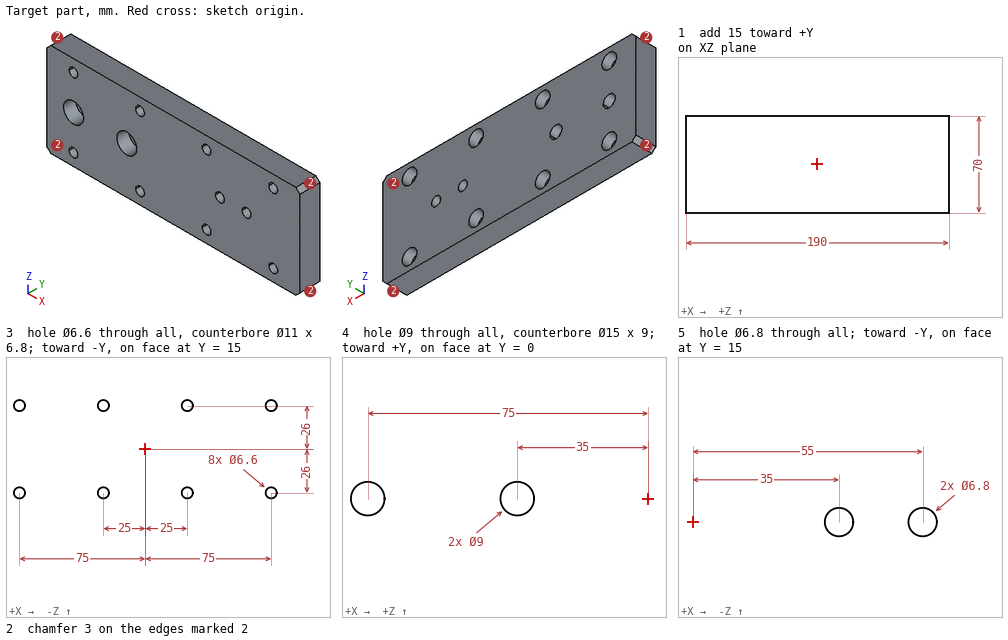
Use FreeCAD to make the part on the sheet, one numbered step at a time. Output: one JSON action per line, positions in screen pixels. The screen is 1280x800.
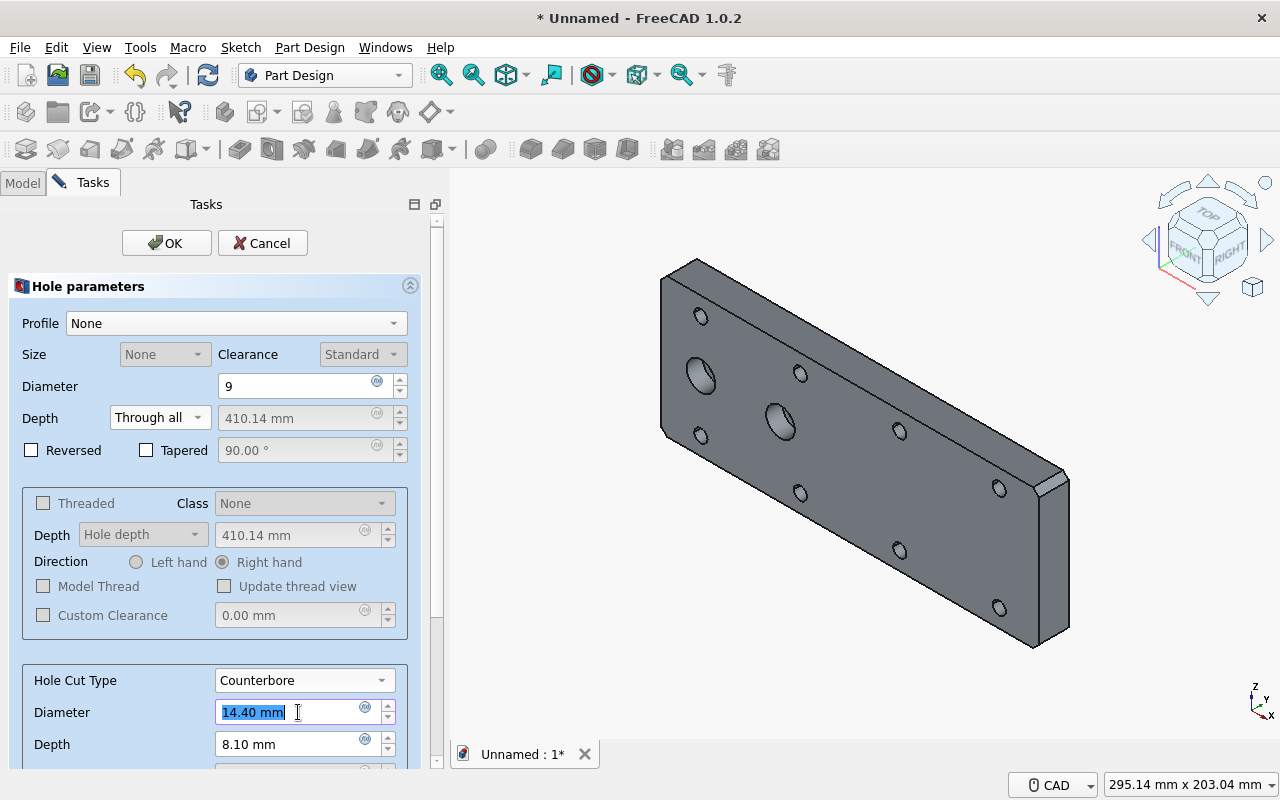
{"action": "type", "text": "15"}
{"action": "key", "text": "Tab"}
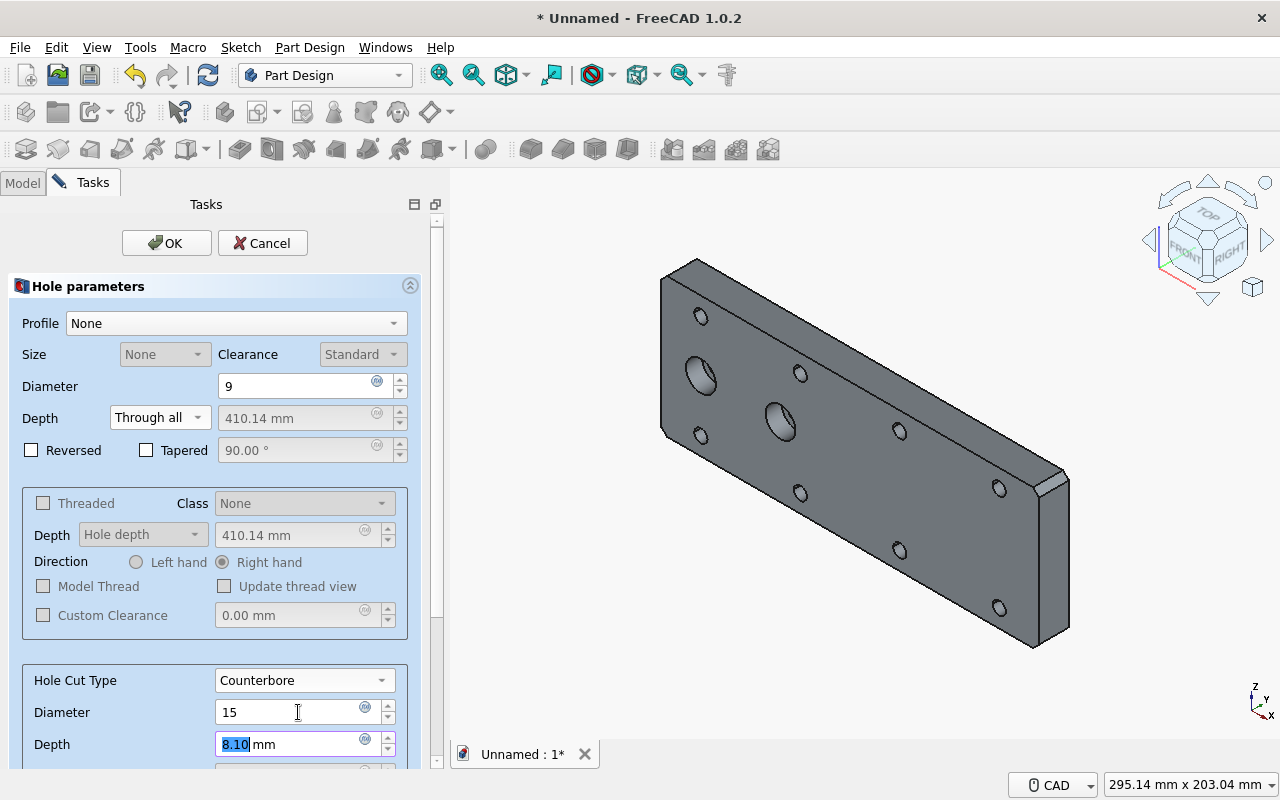
{"action": "type", "text": "9"}
{"action": "key", "text": "Tab"}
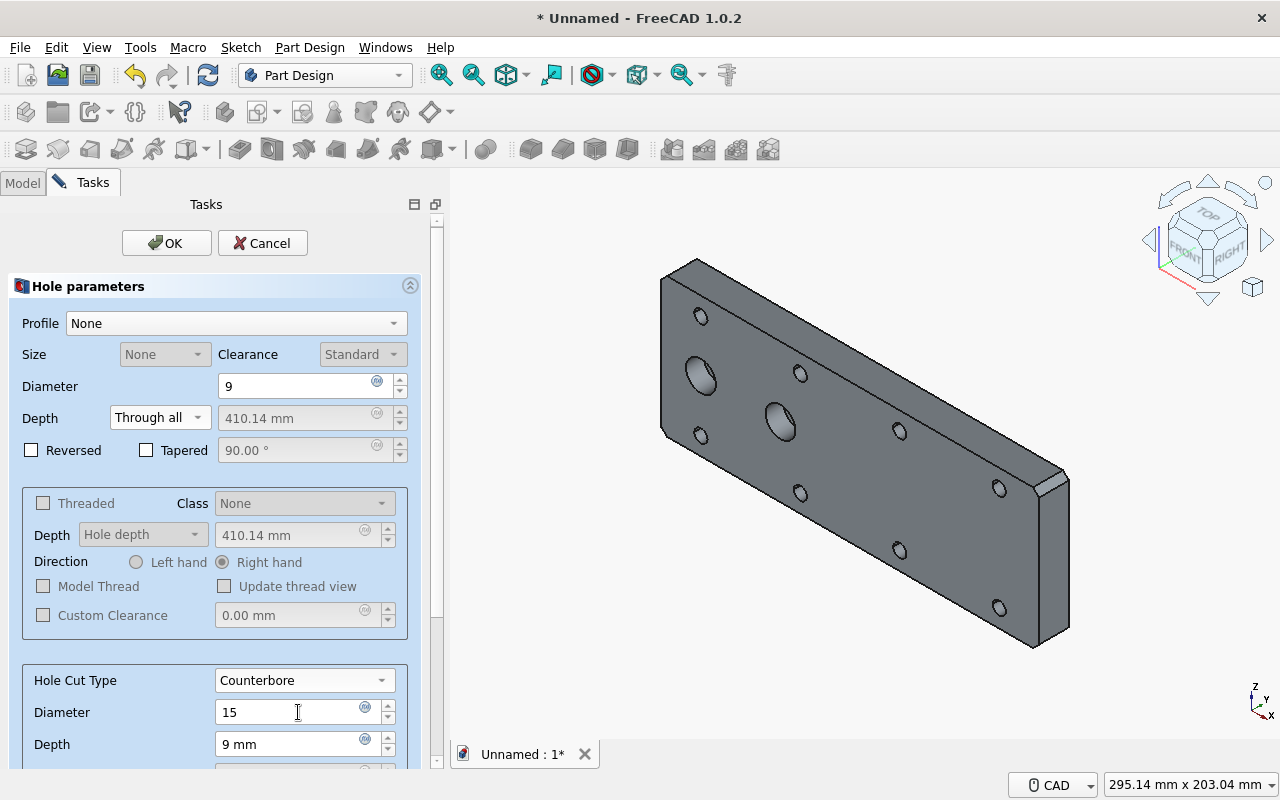
{"action": "left_click", "coordinate": [167, 243]}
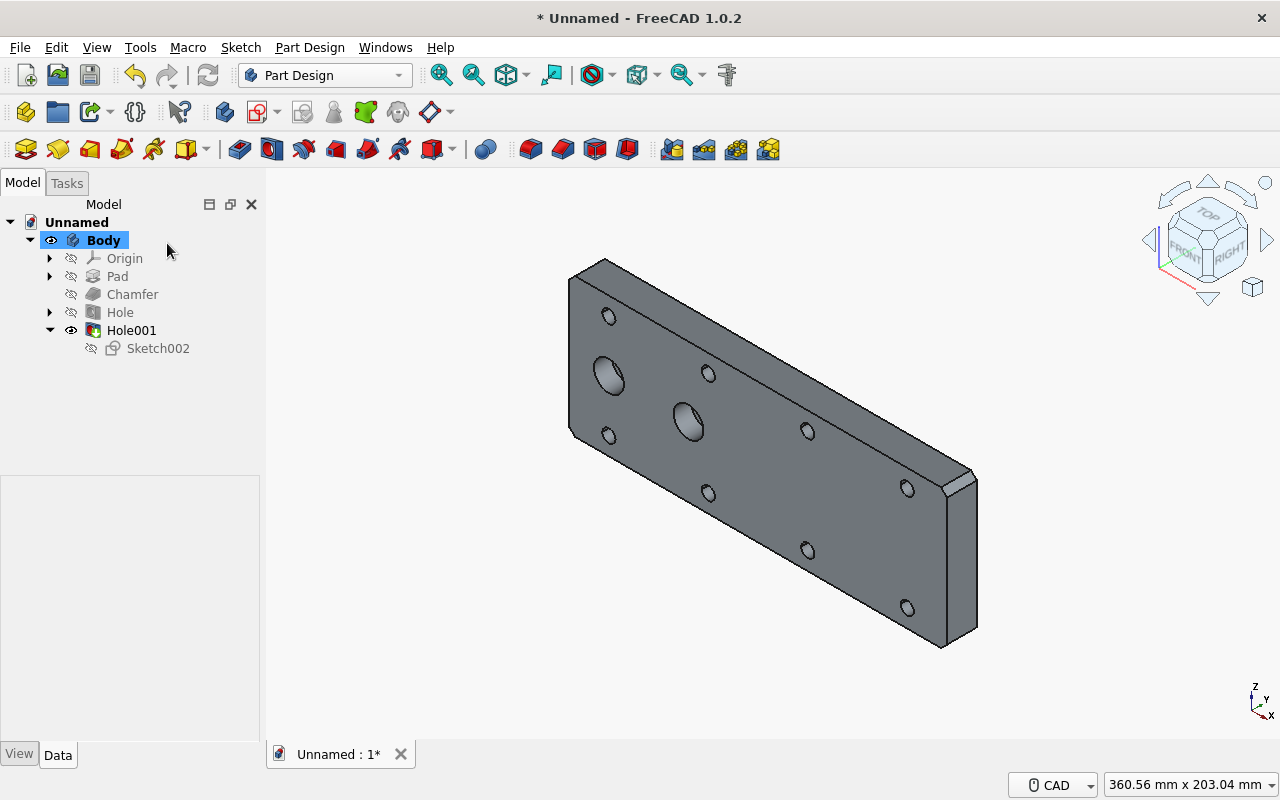
{"action": "key", "text": "4"}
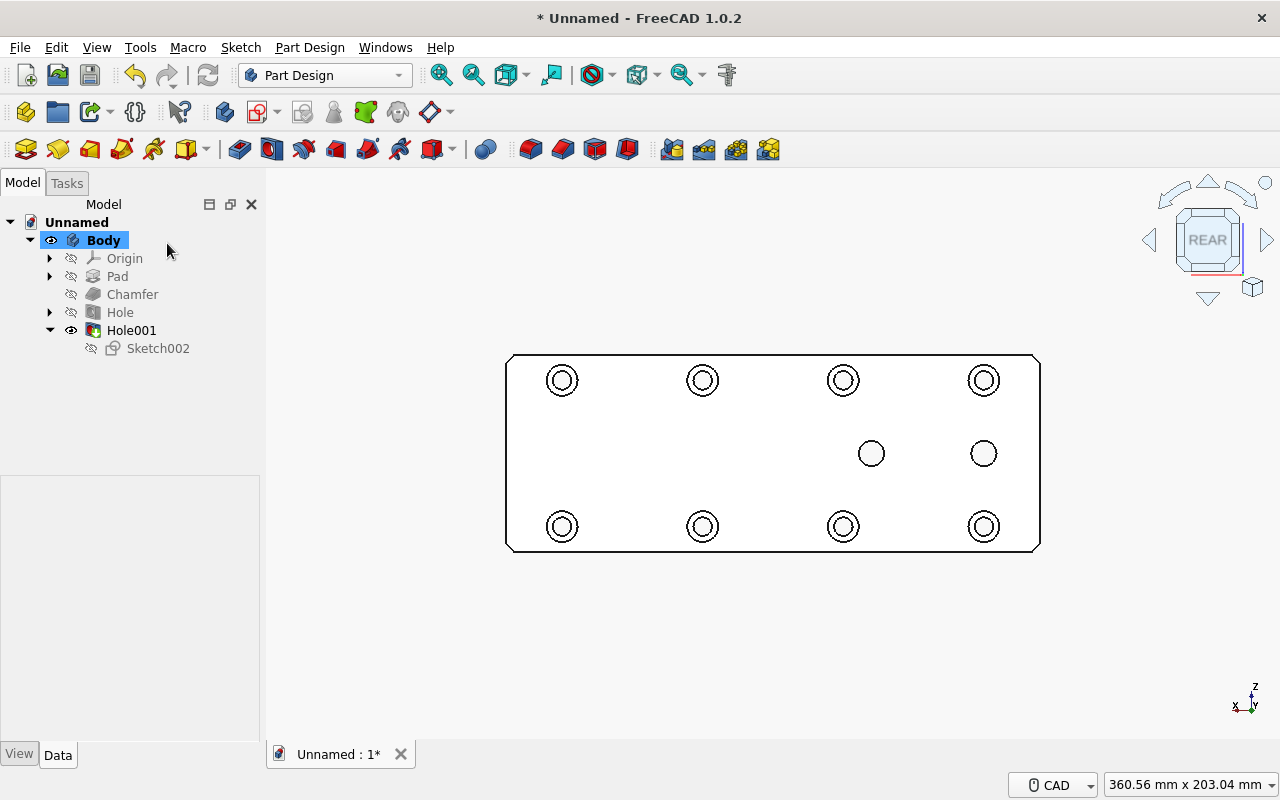
{"action": "left_click", "coordinate": [773, 453]}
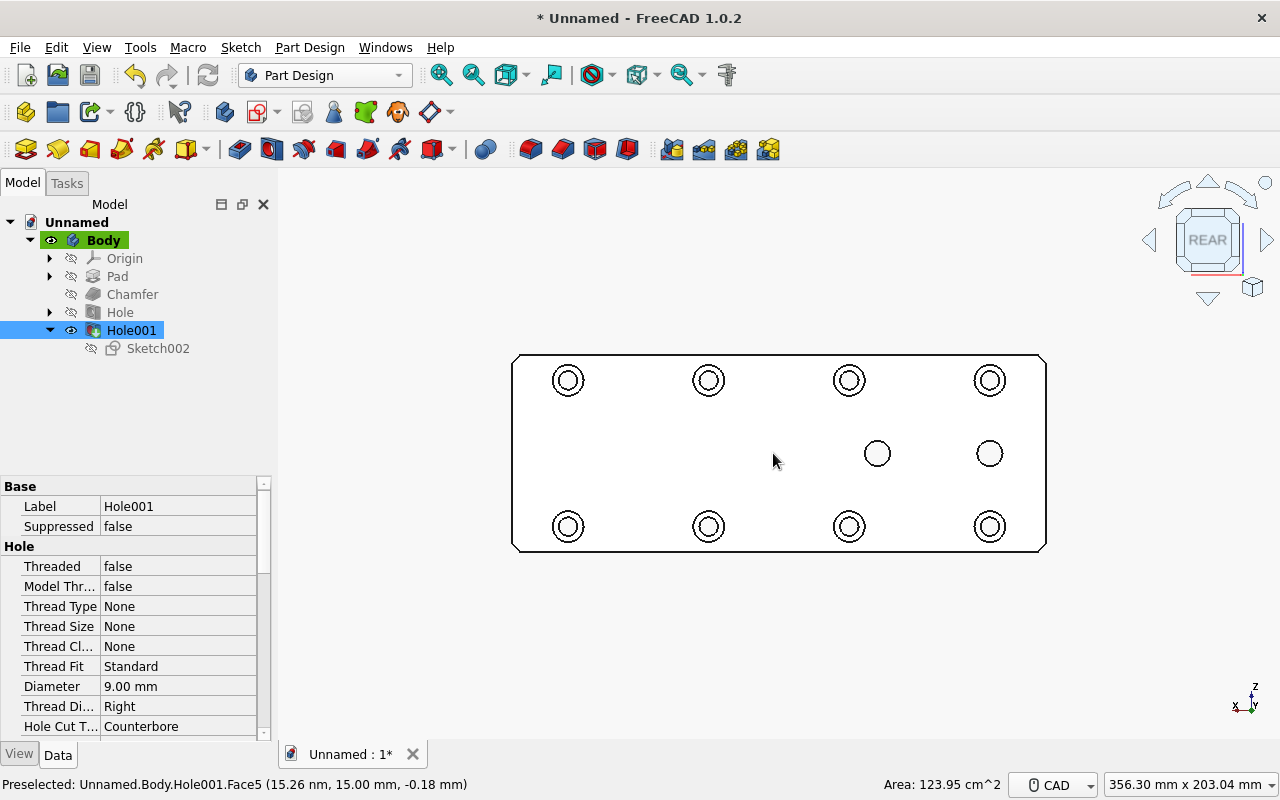
{"action": "left_click", "coordinate": [258, 112]}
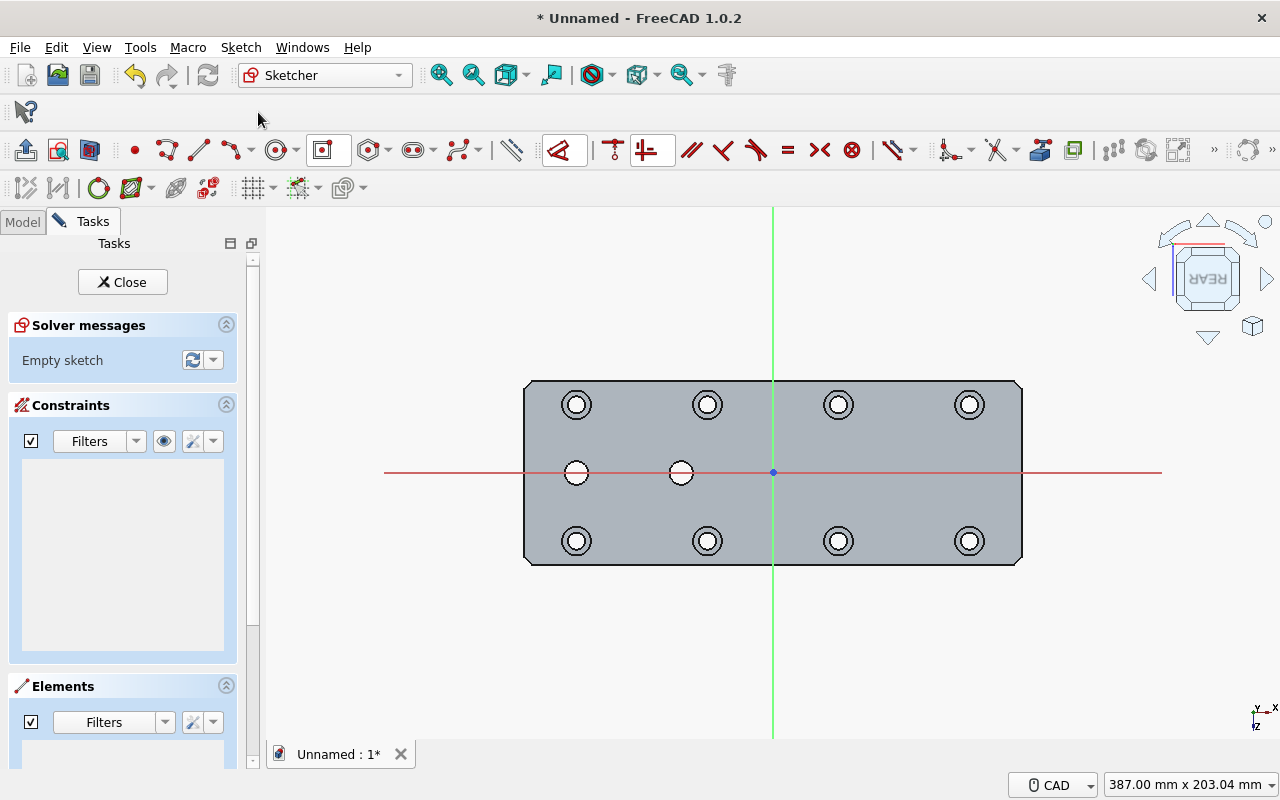
{"action": "scroll", "coordinate": [897, 473], "scroll_direction": "up", "scroll_amount": 7}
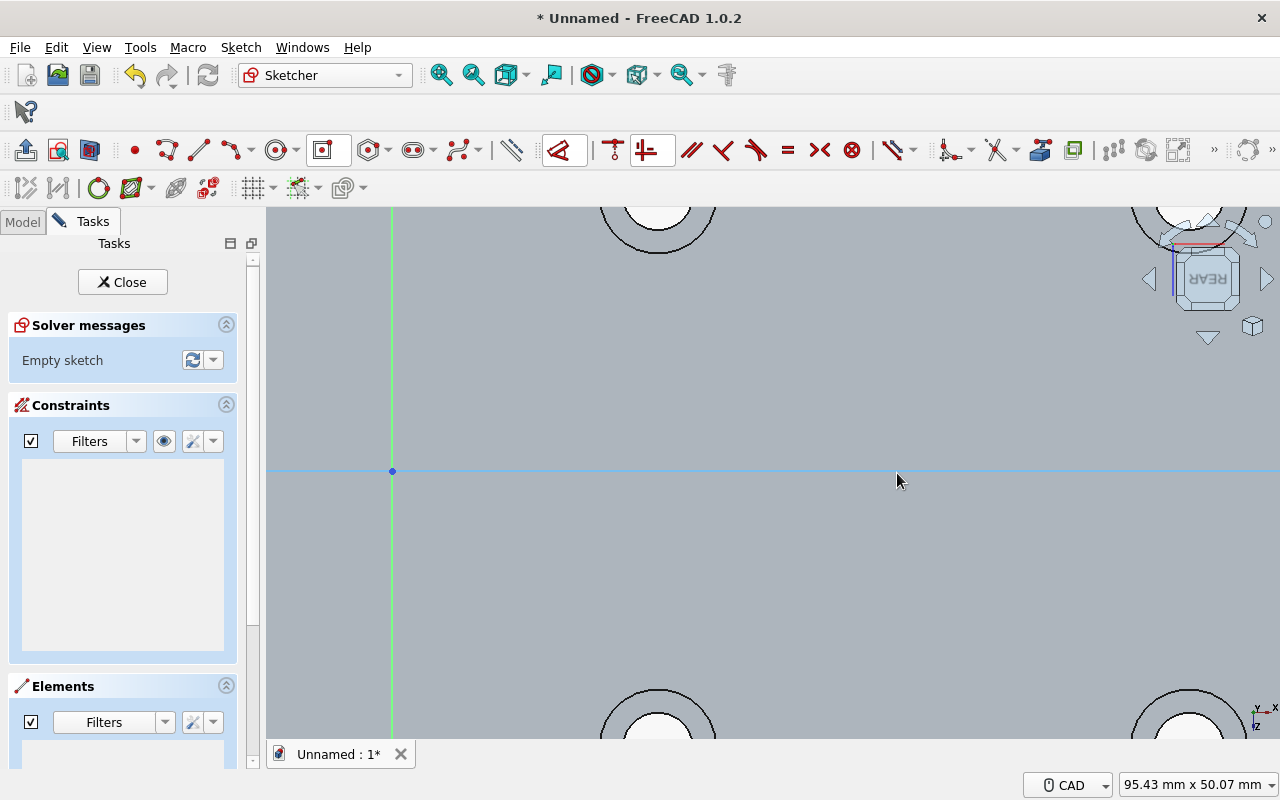
{"action": "key", "text": "g c"}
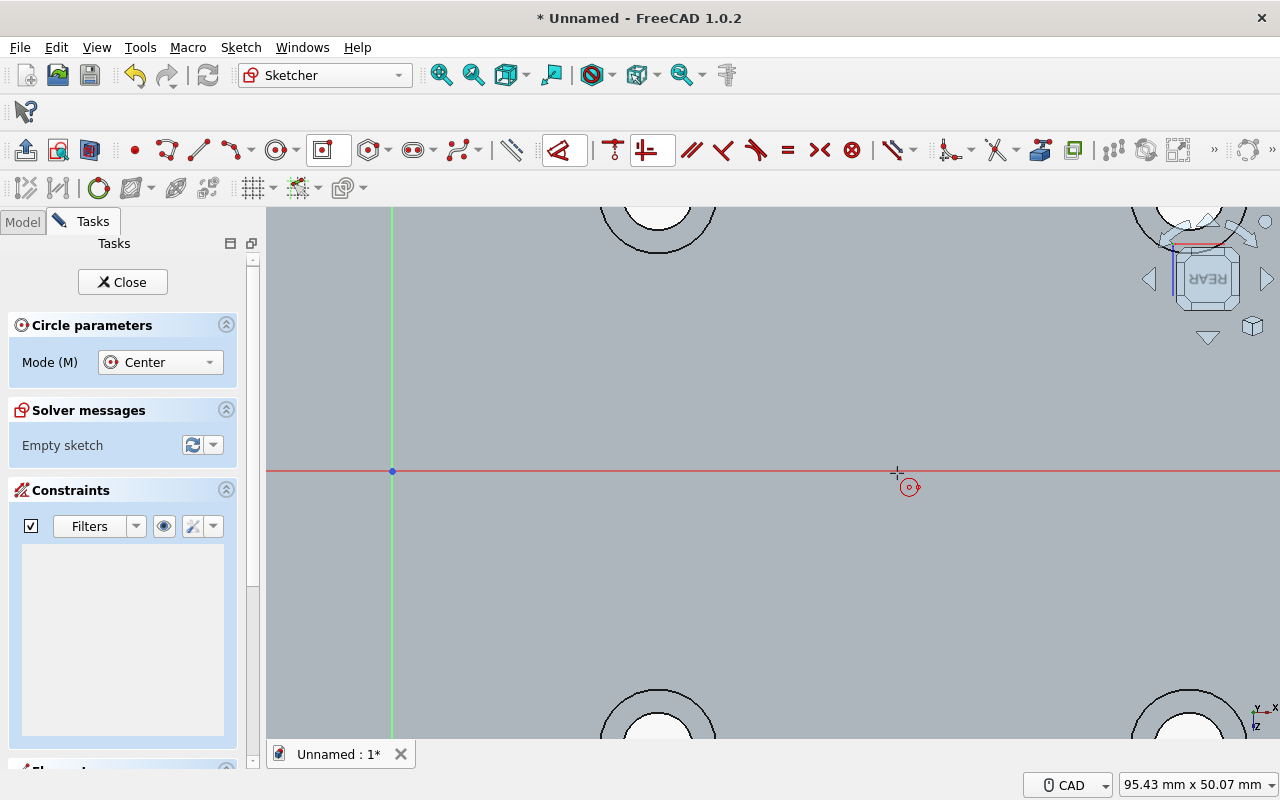
{"action": "left_click", "coordinate": [977, 471]}
{"action": "mouse_move", "coordinate": [1002, 446]}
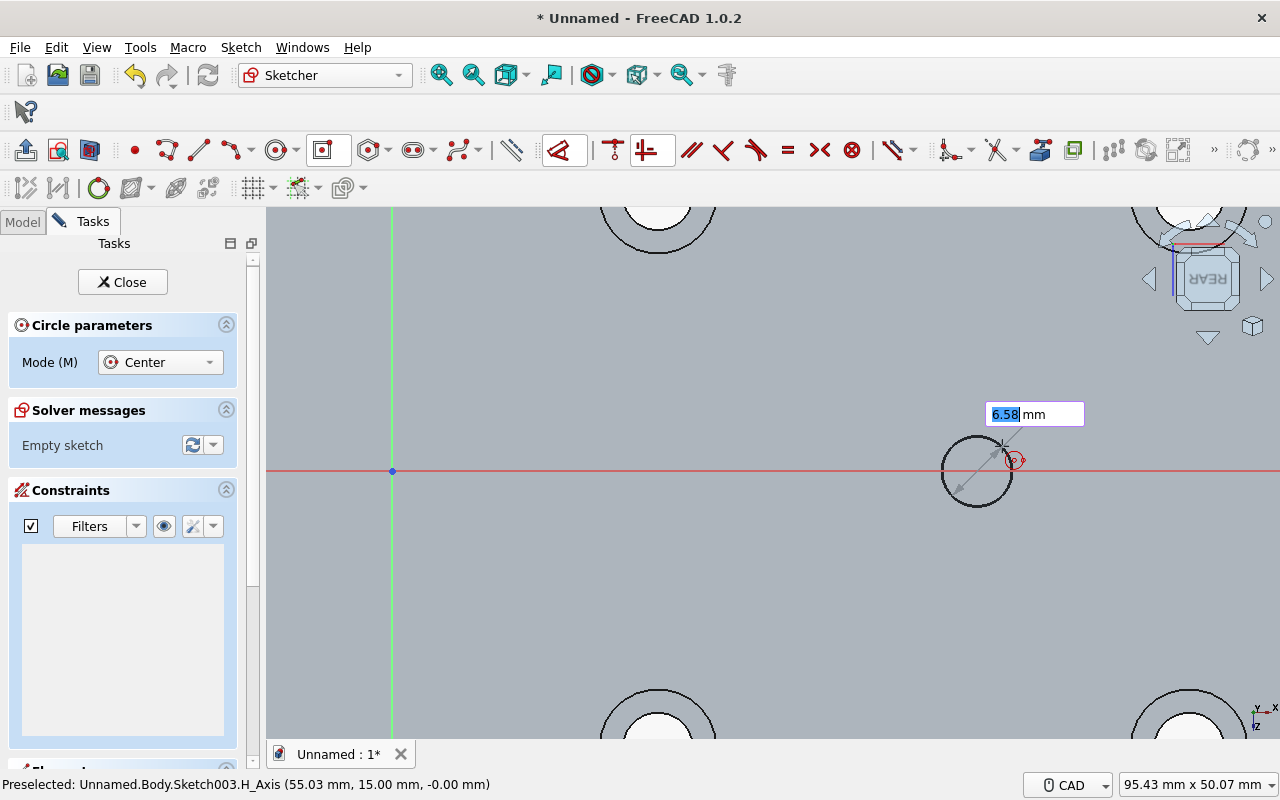
{"action": "type", "text": "6.8"}
{"action": "key", "text": "Return"}